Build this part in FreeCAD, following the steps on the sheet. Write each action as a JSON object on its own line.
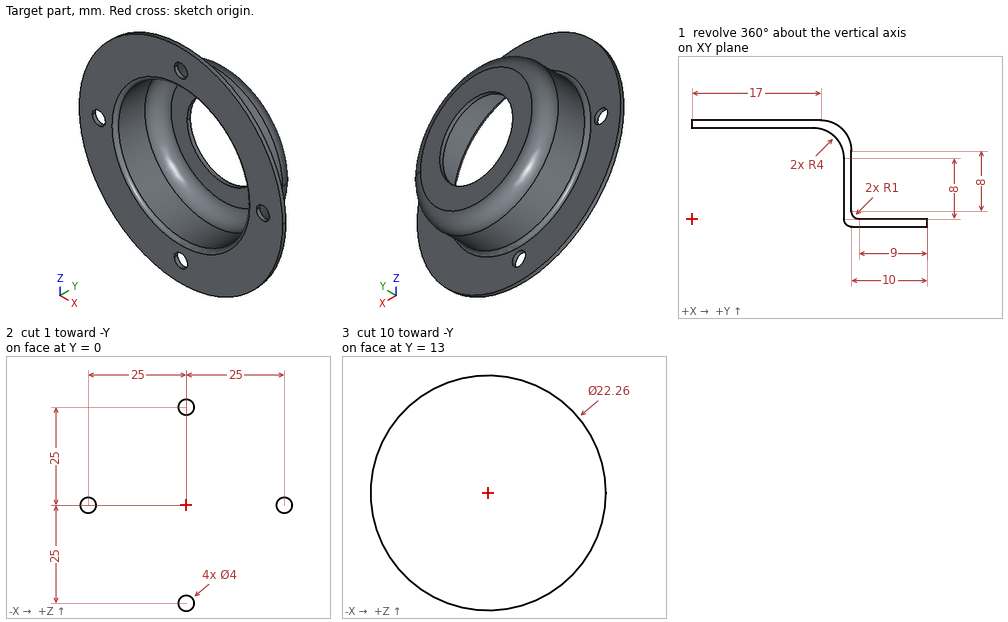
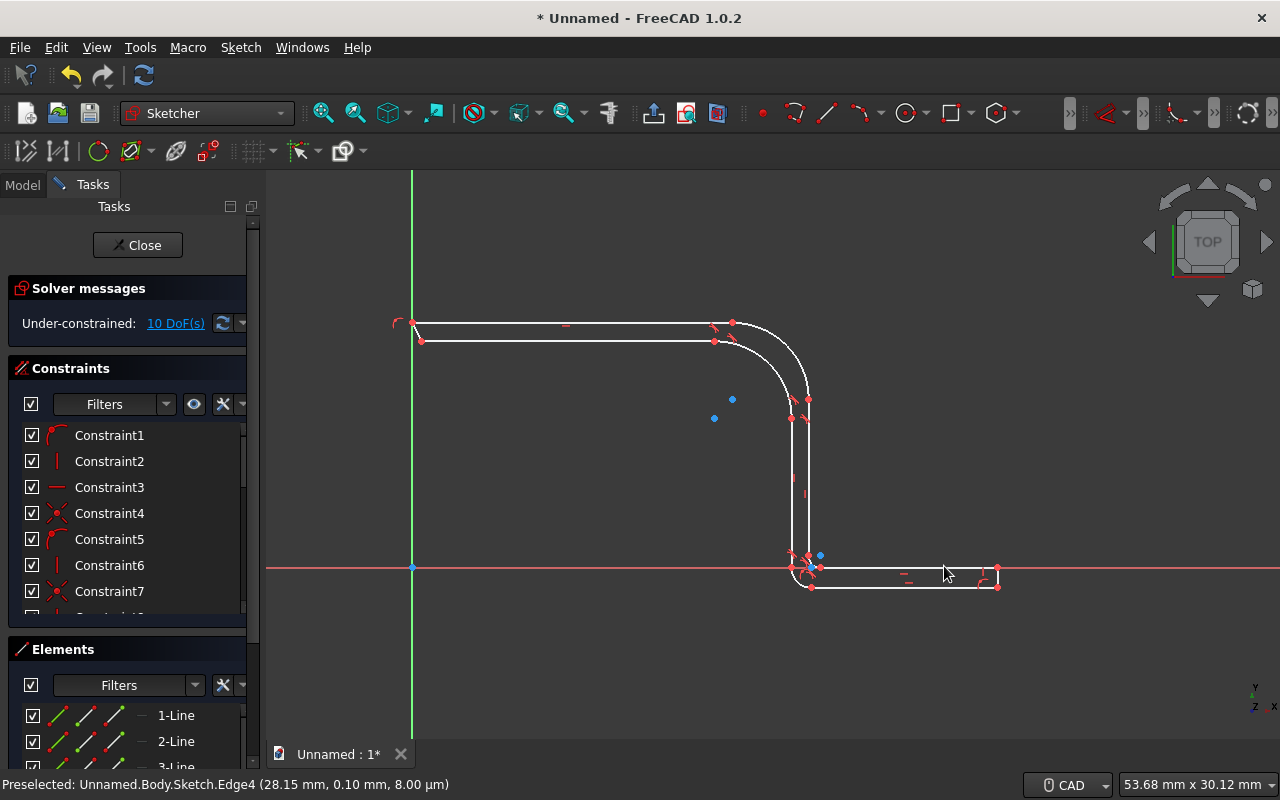
{"action": "scroll", "coordinate": [416, 330], "scroll_direction": "up", "scroll_amount": 4}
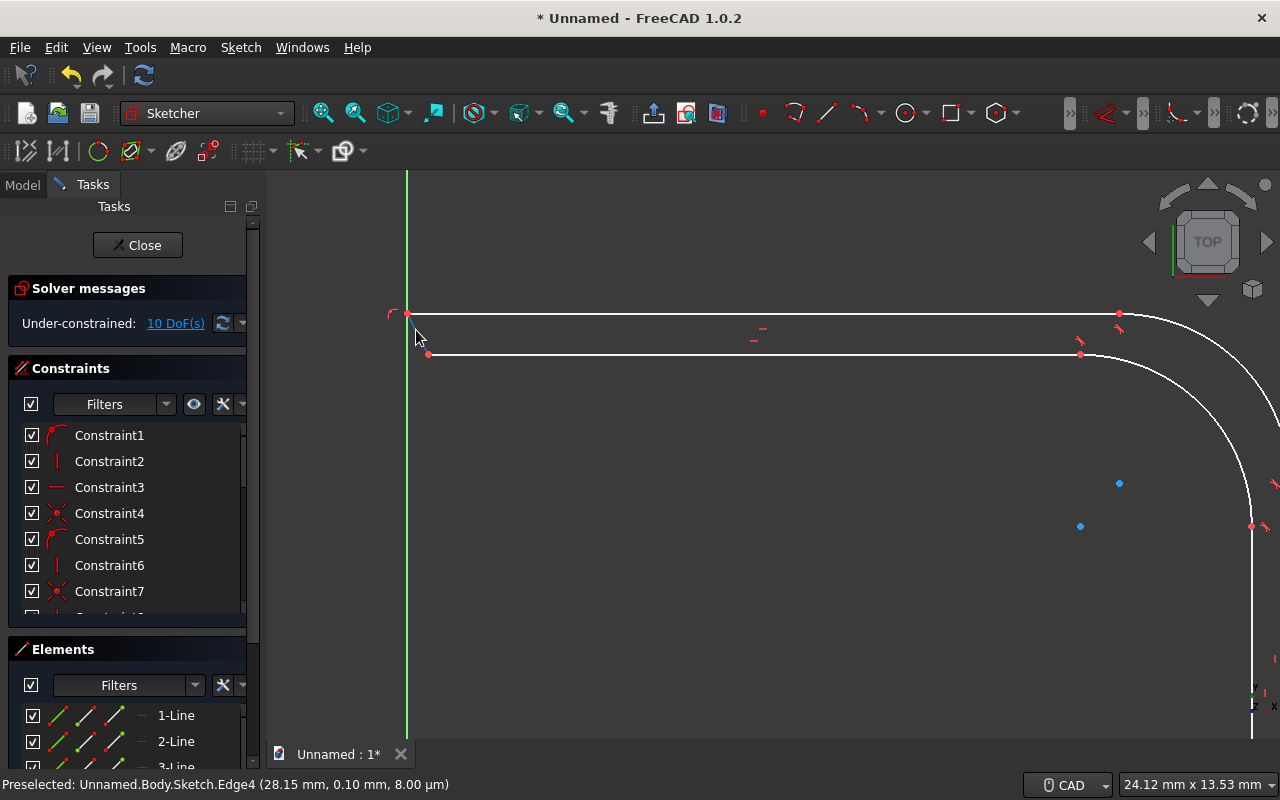
{"action": "left_click", "coordinate": [416, 330]}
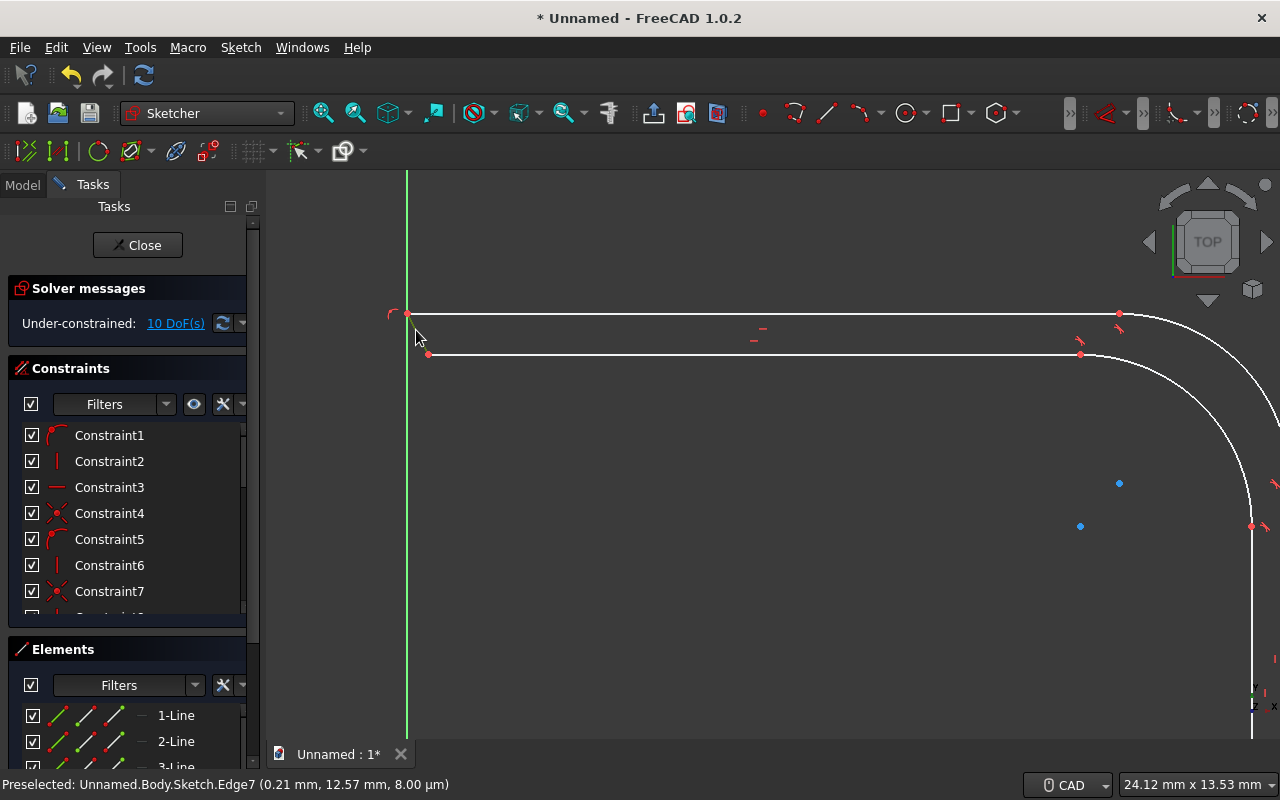
{"action": "key", "text": "v"}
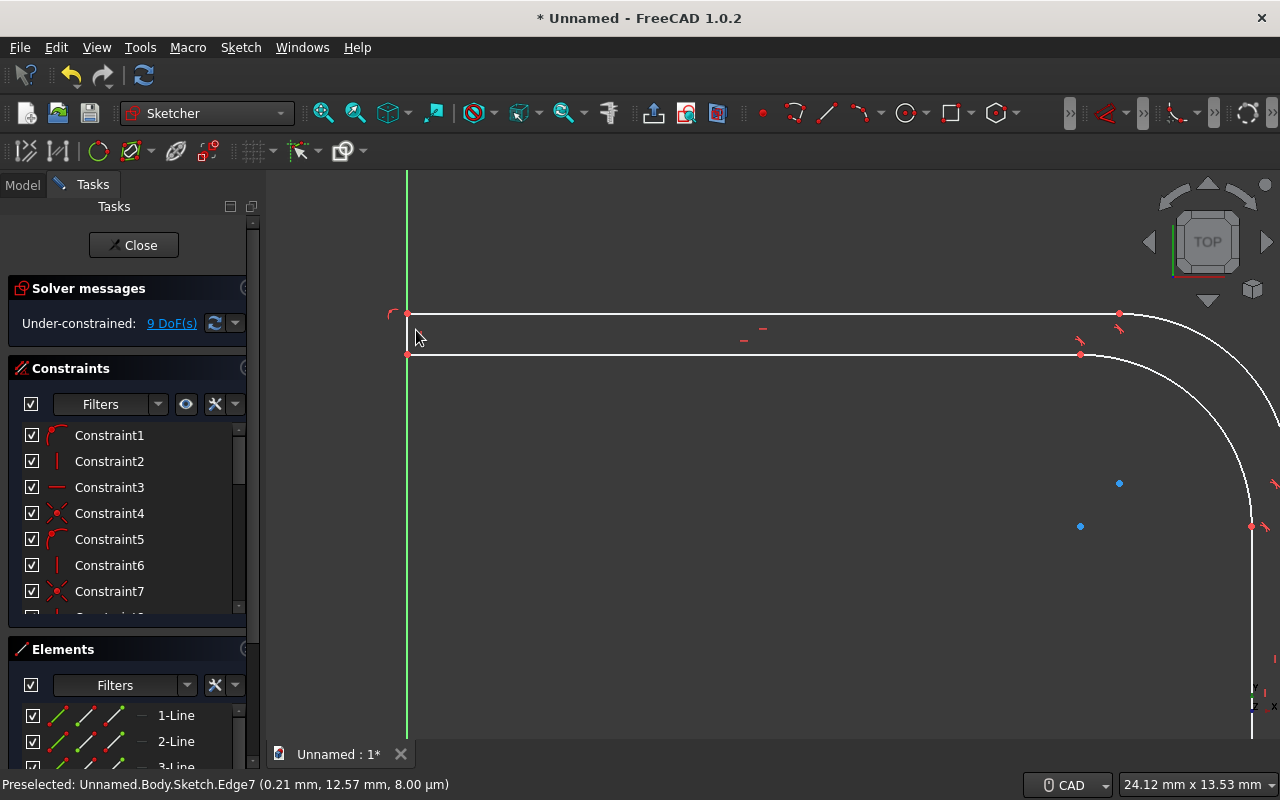
{"action": "scroll", "coordinate": [415, 330], "scroll_direction": "down", "scroll_amount": 4}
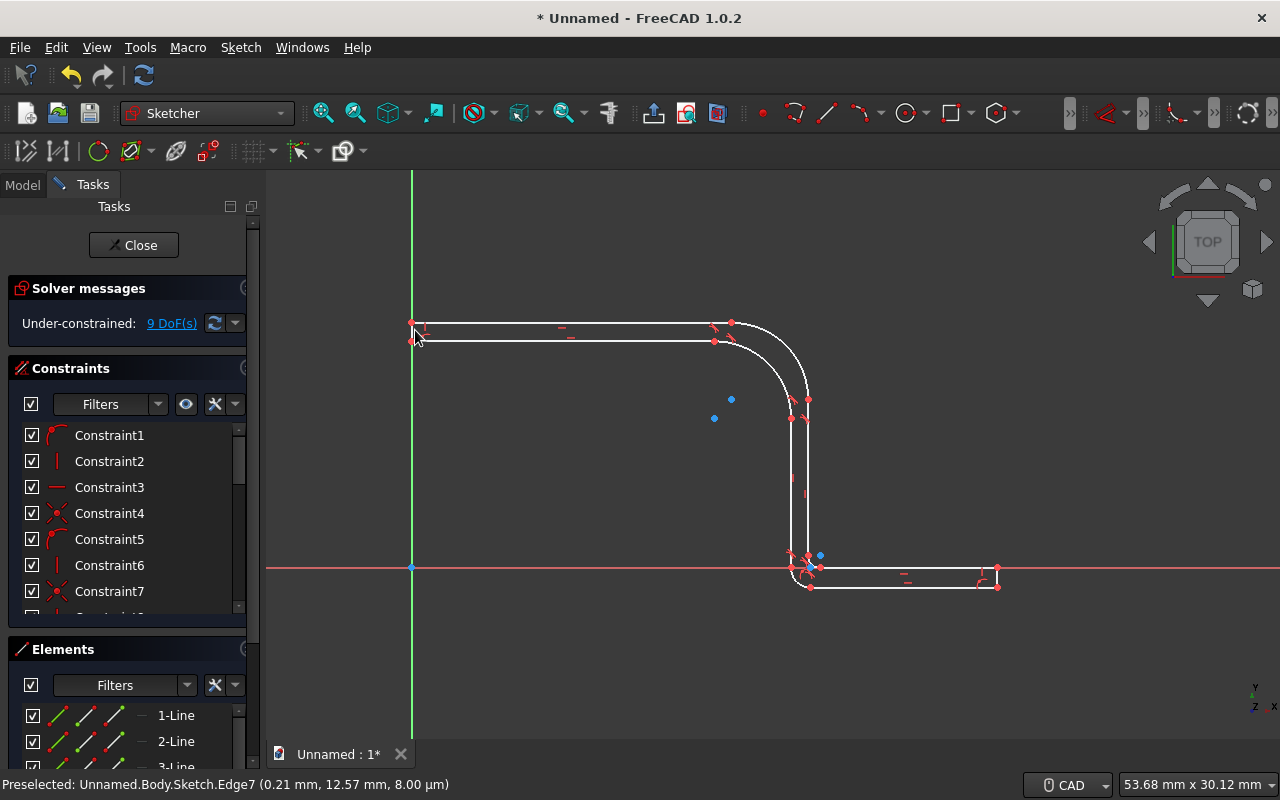
{"action": "scroll", "coordinate": [793, 577], "scroll_direction": "up", "scroll_amount": 3}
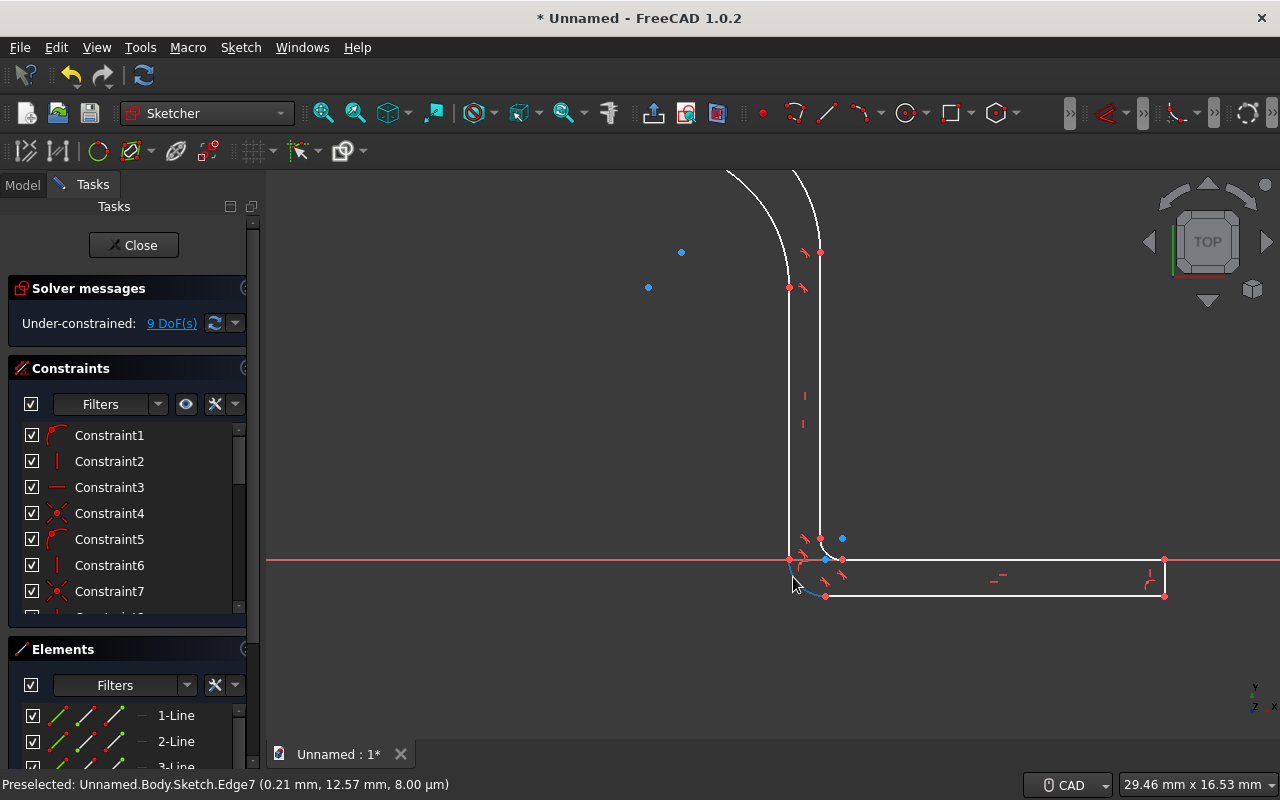
{"action": "left_click", "coordinate": [793, 576]}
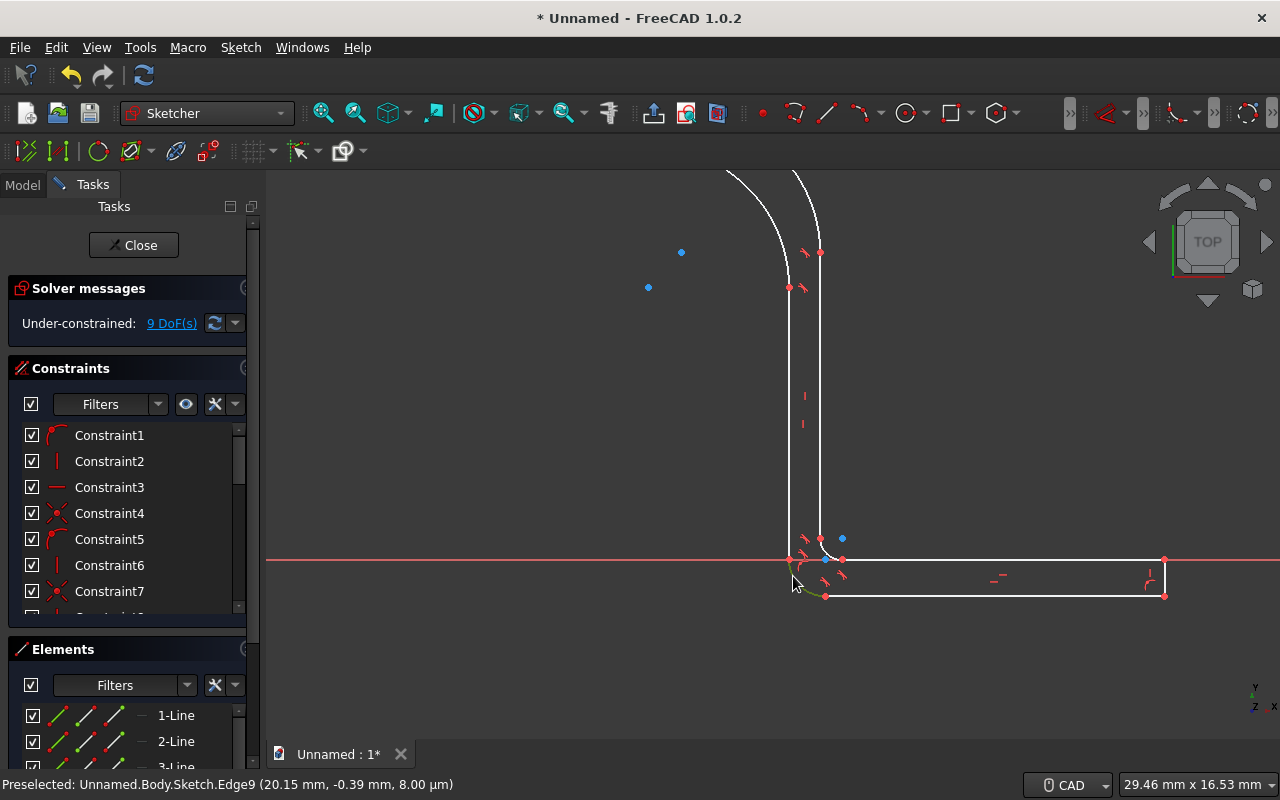
{"action": "scroll", "coordinate": [823, 548], "scroll_direction": "up", "scroll_amount": 2}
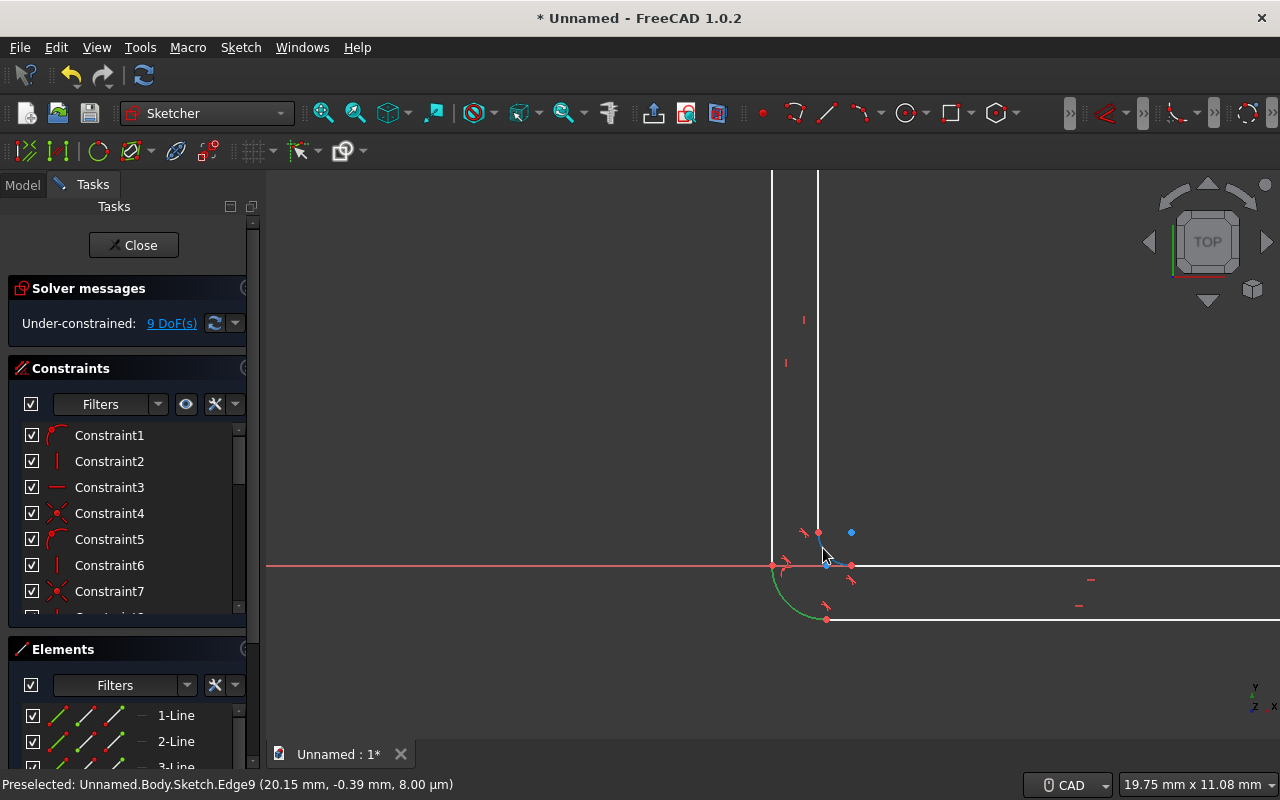
{"action": "left_click", "coordinate": [822, 548]}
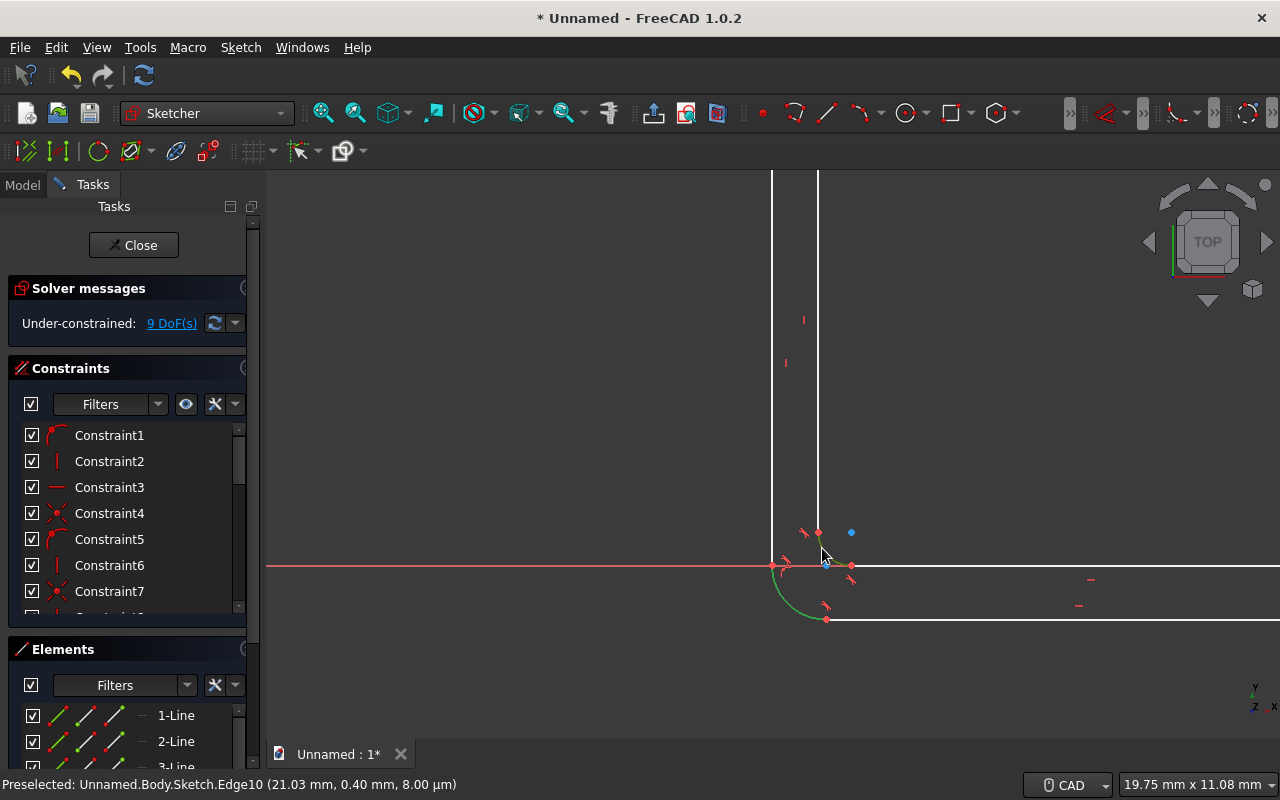
{"action": "key", "text": "e"}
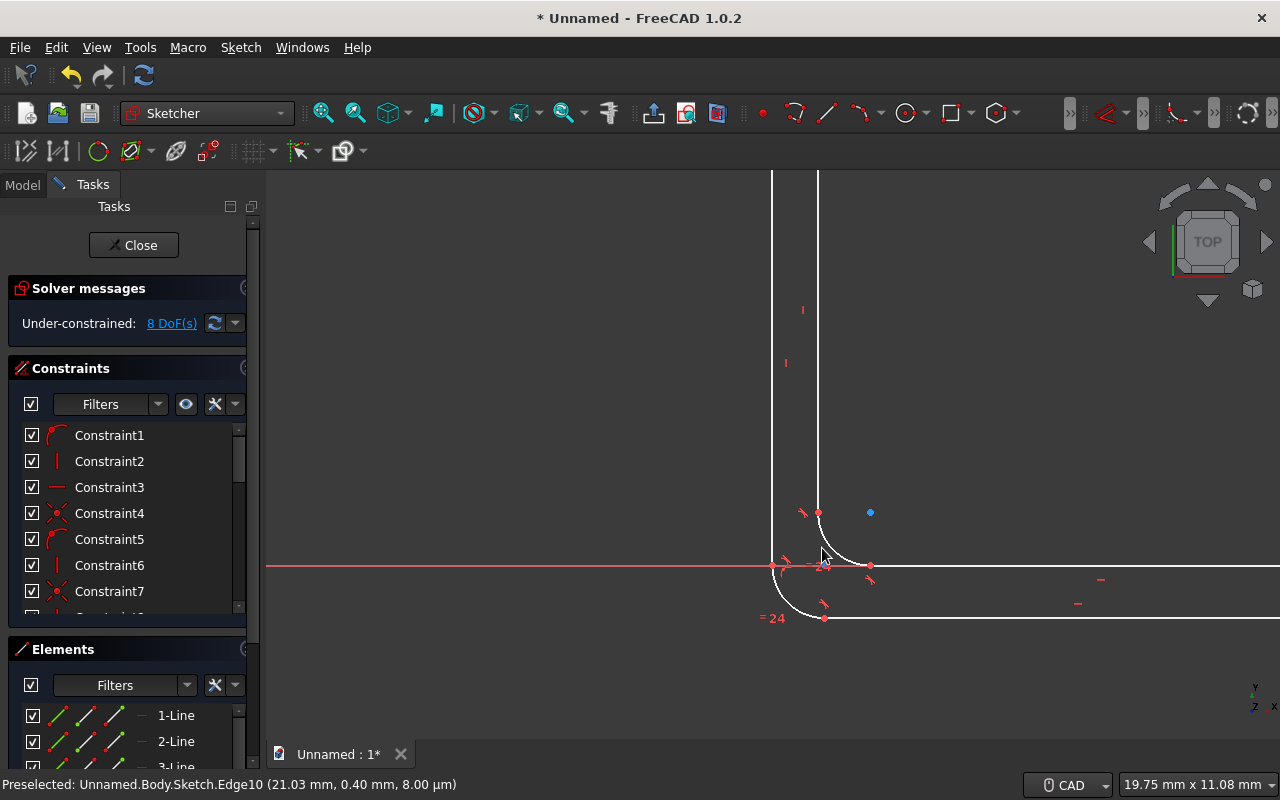
{"action": "scroll", "coordinate": [802, 569], "scroll_direction": "down", "scroll_amount": 5}